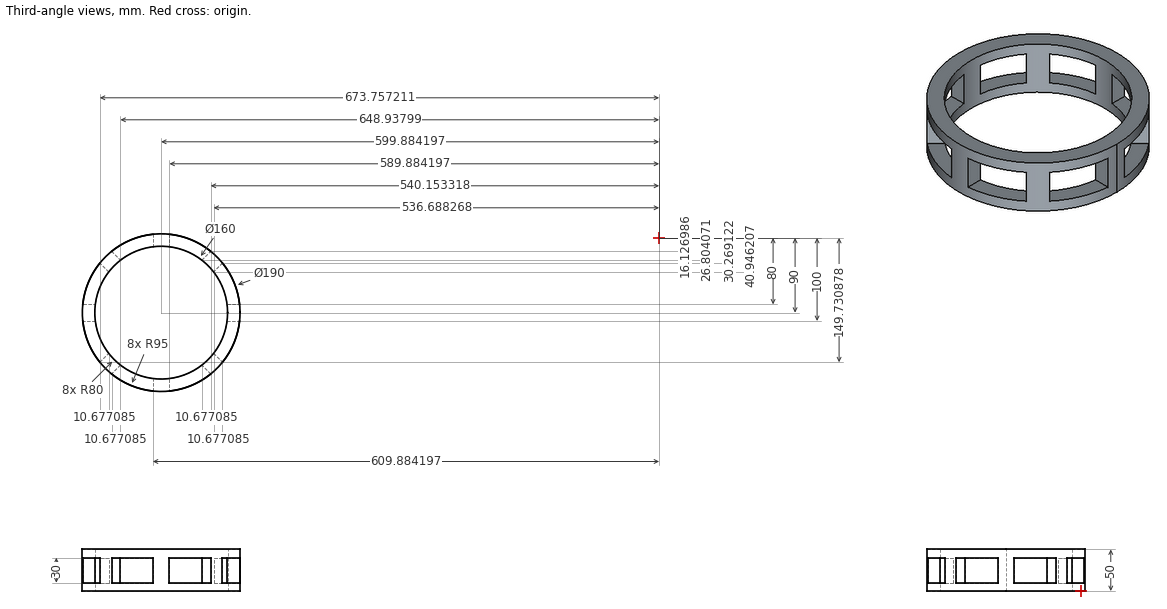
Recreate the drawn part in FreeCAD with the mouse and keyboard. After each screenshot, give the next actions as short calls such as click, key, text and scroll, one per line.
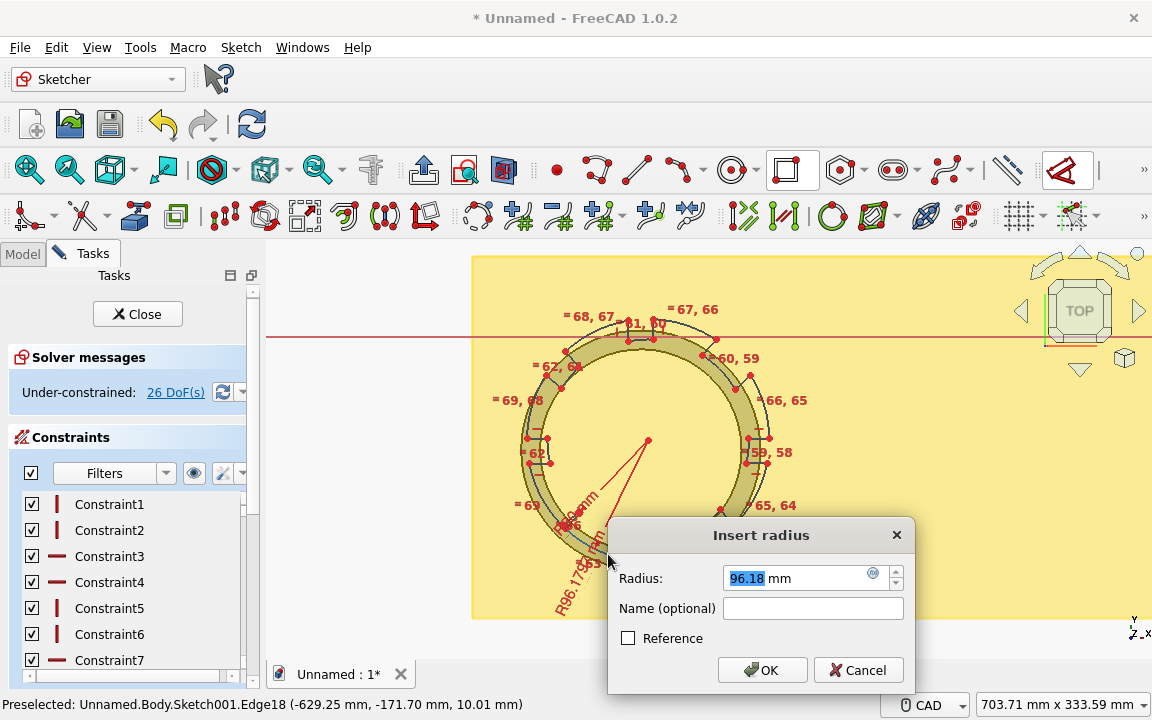
text(95)
key(Return)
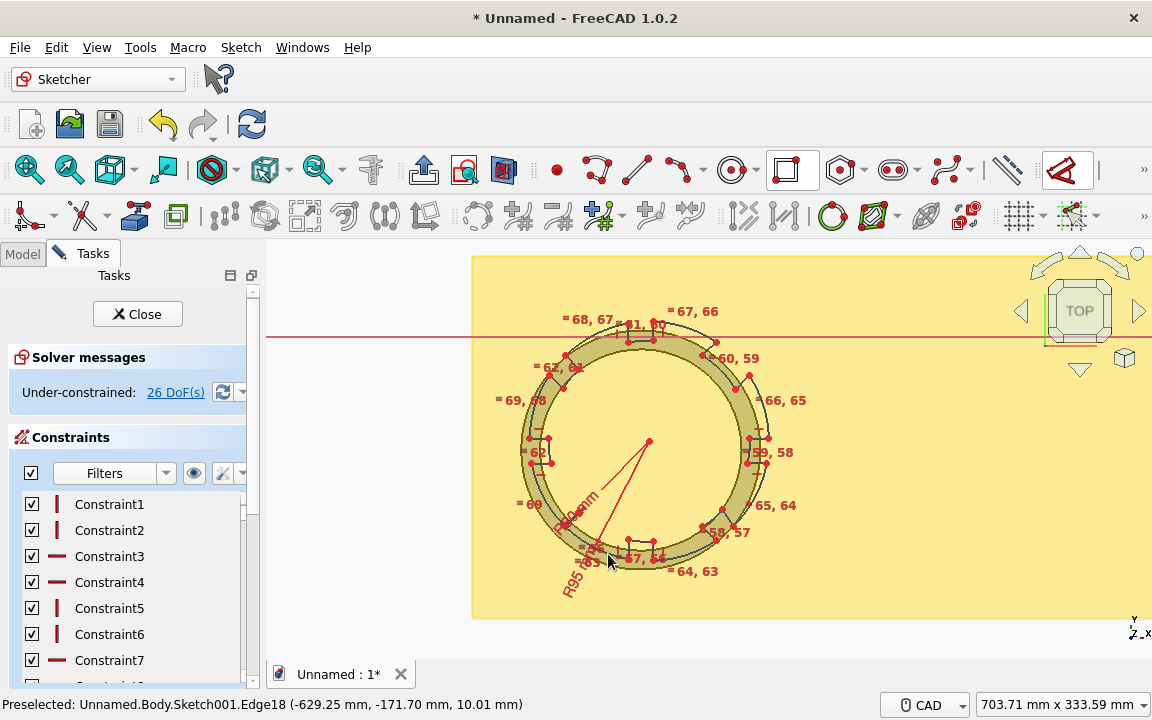
click(750, 439)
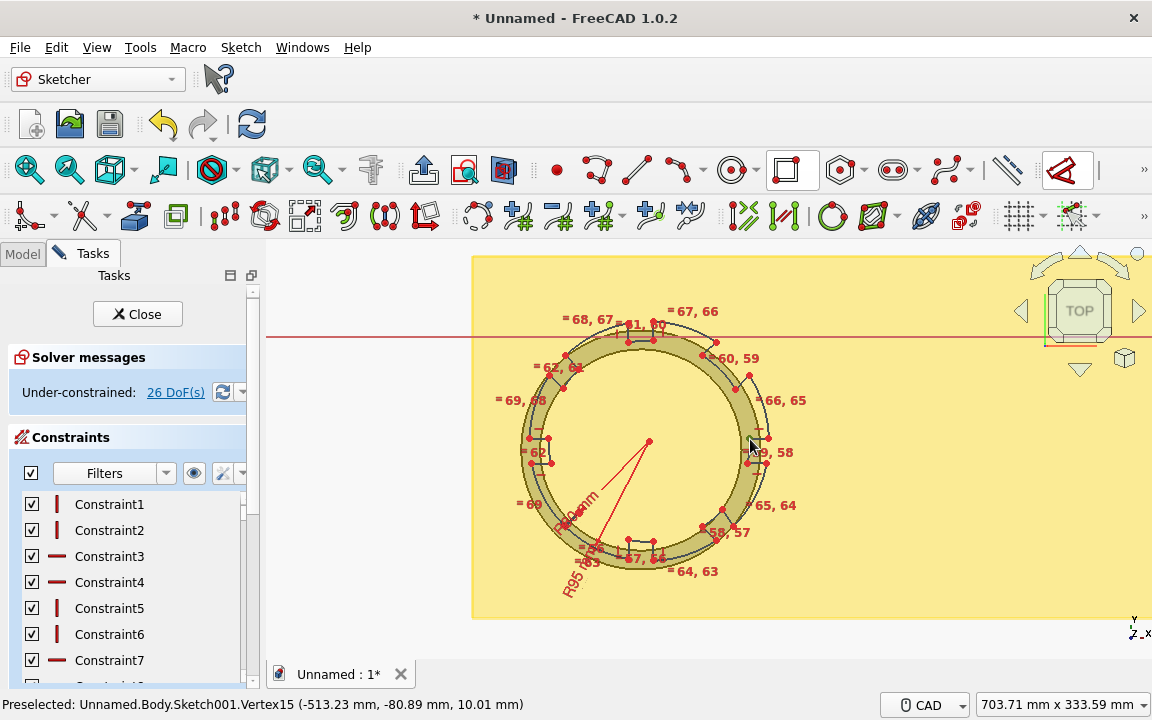
key(i)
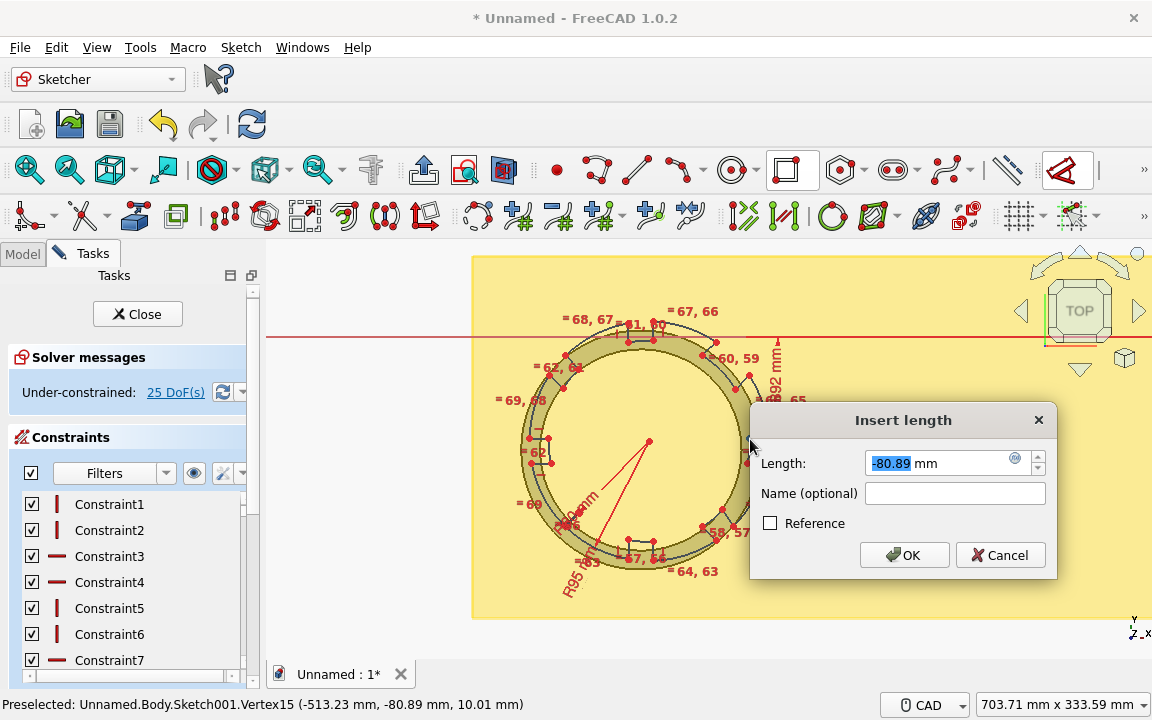
text(-80)
key(Return)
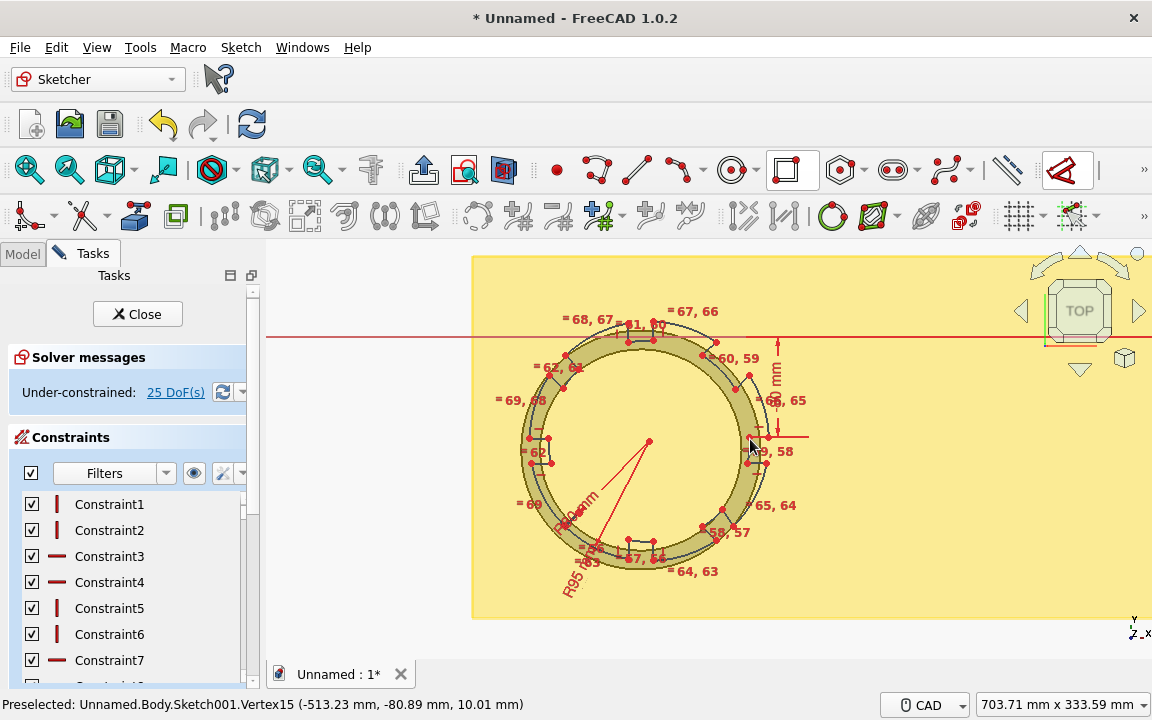
click(530, 439)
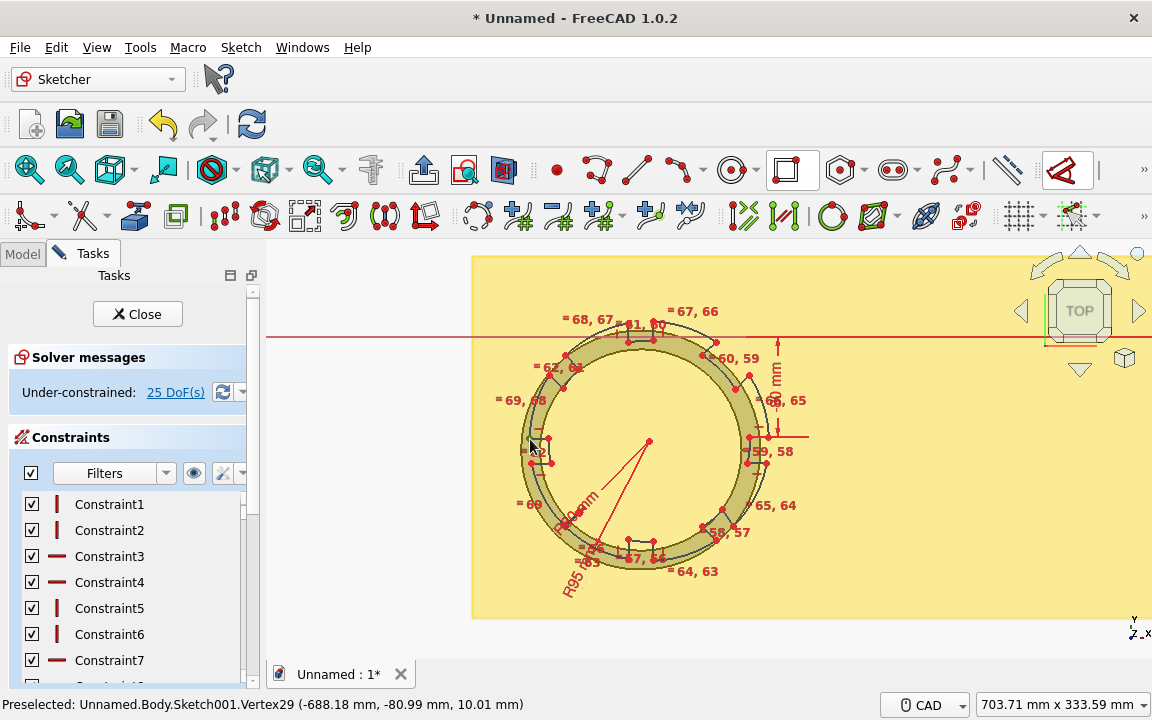
key(i)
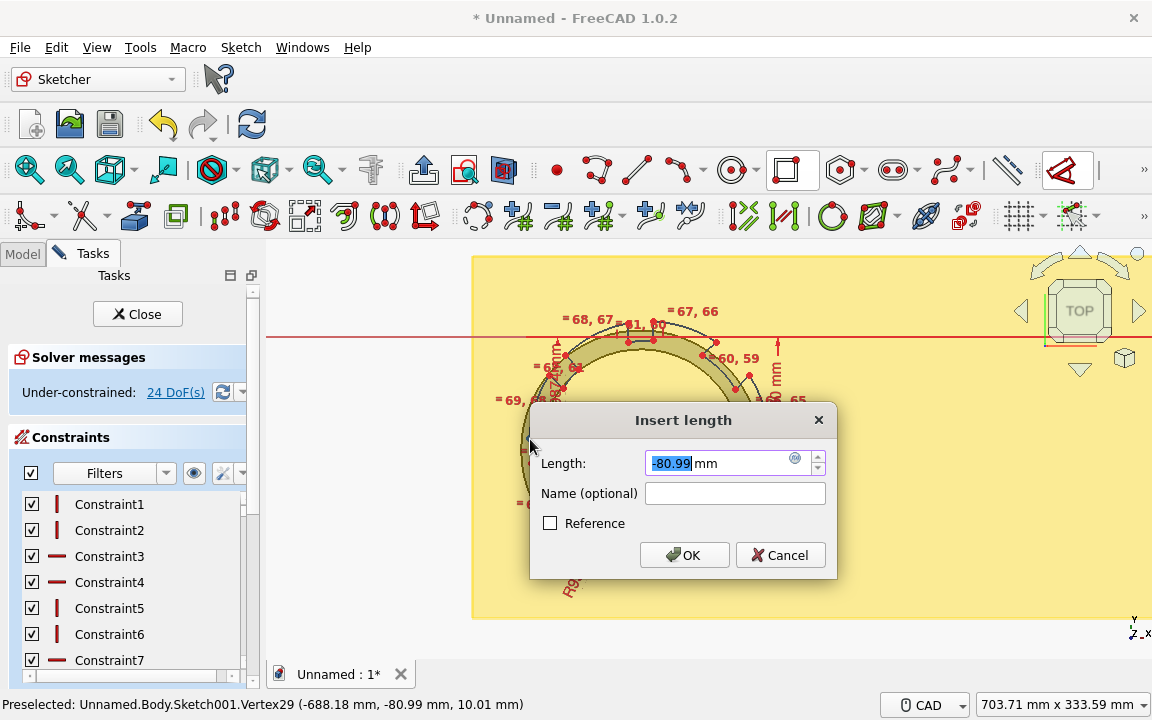
text(-80)
key(Return)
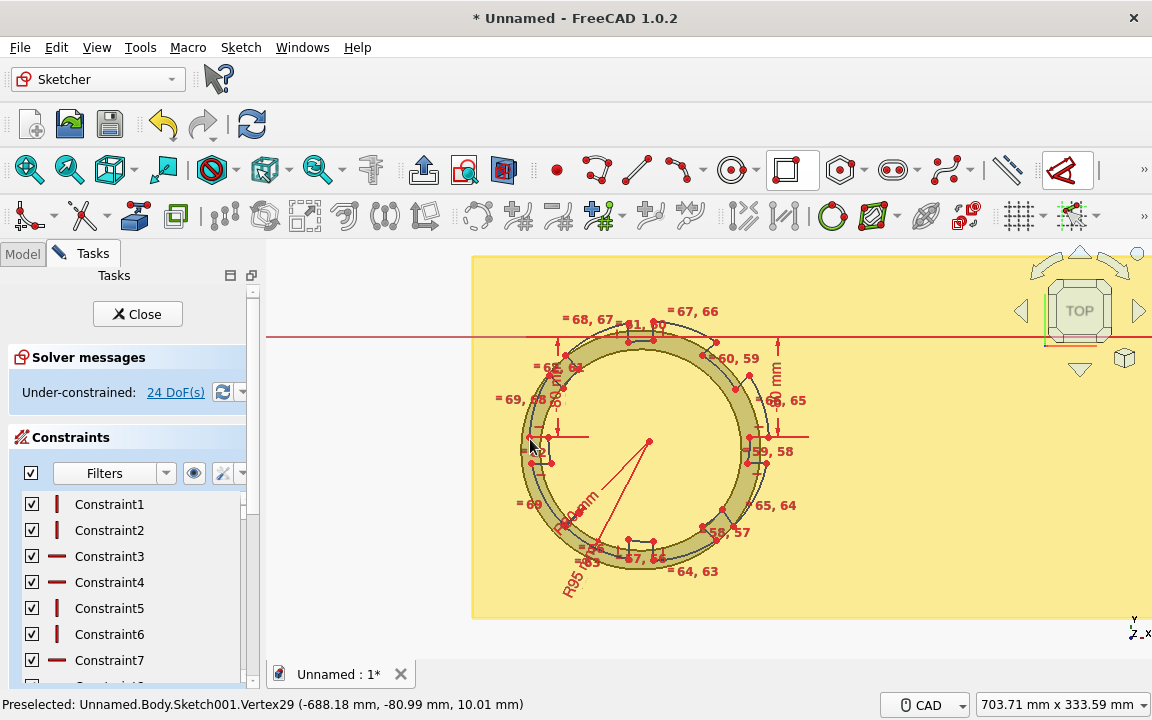
click(649, 441)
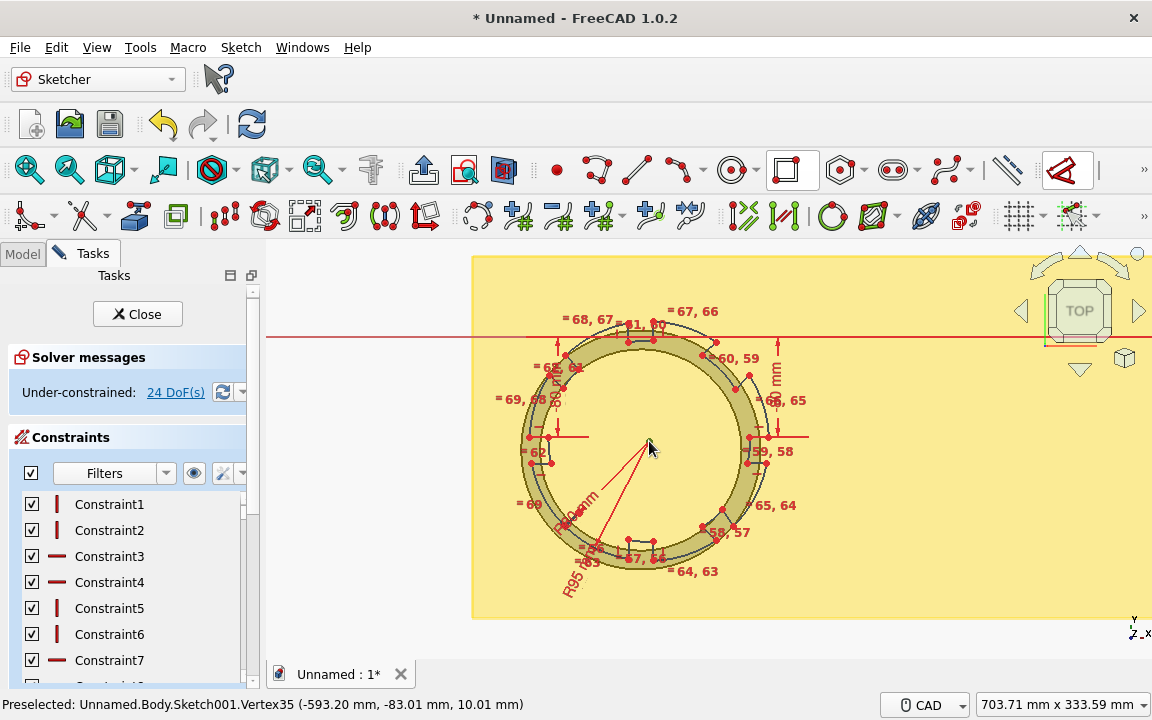
key(i)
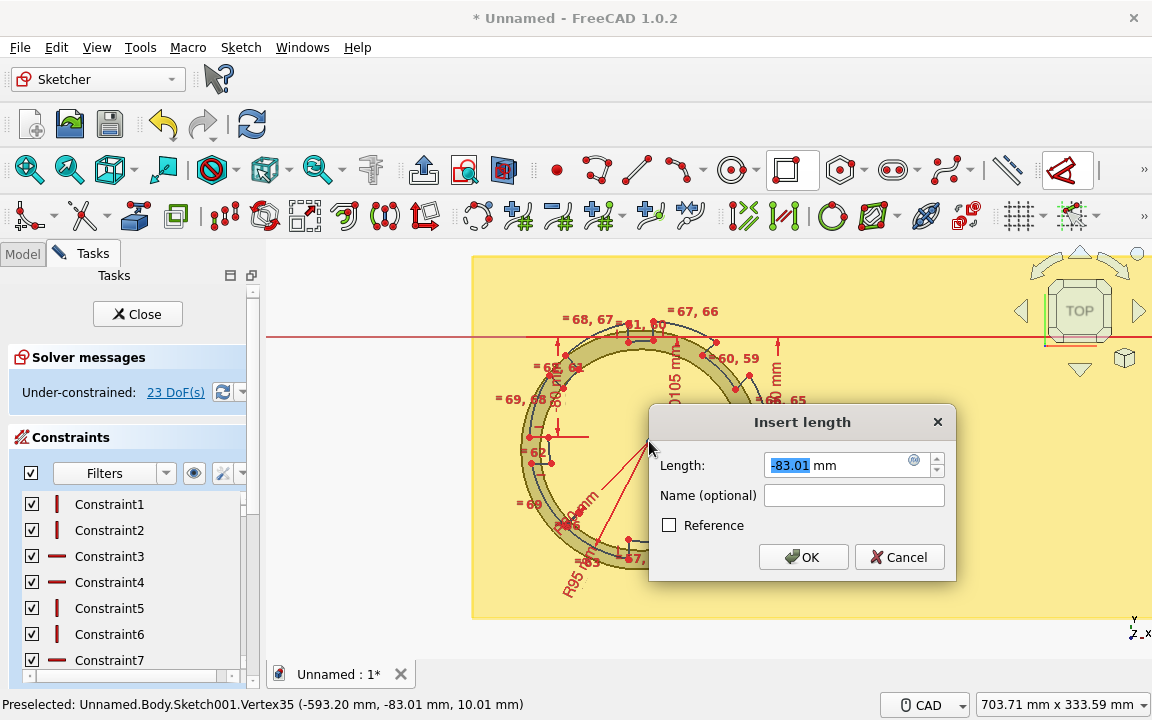
text(-90)
key(Return)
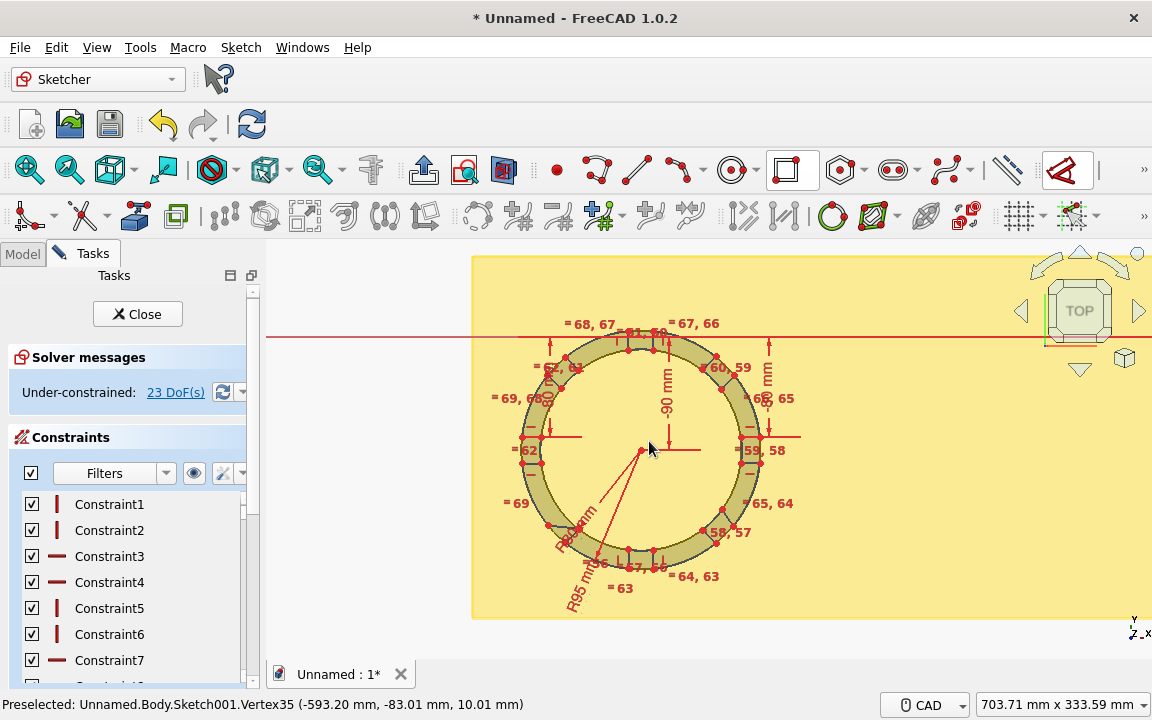
click(760, 463)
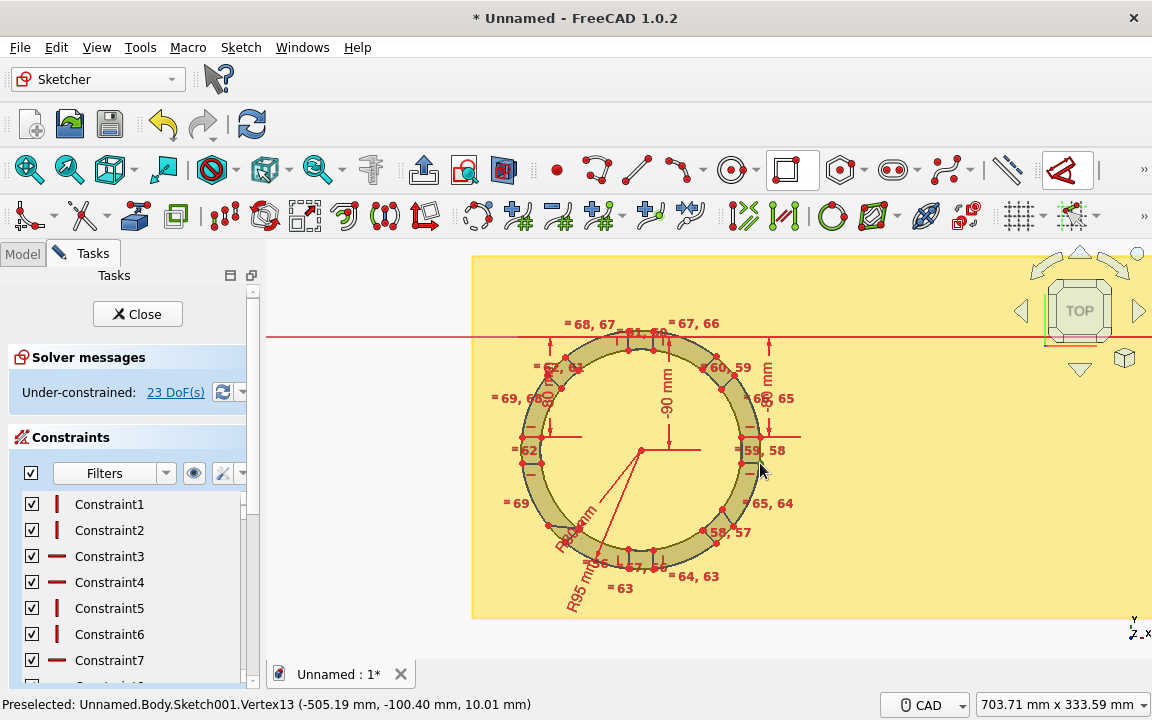
key(i)